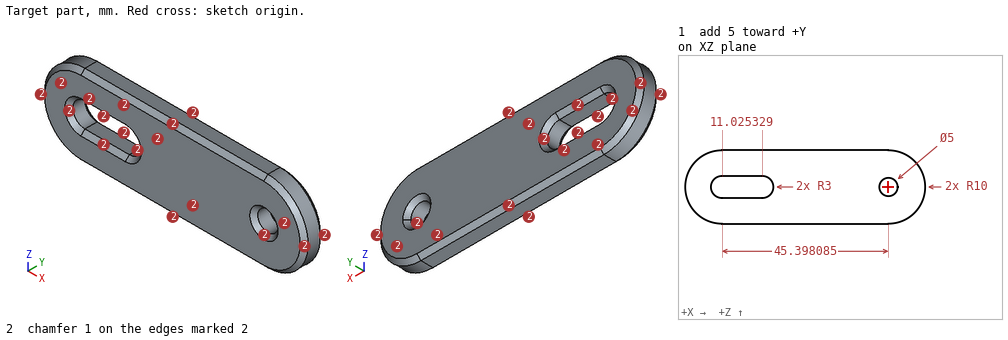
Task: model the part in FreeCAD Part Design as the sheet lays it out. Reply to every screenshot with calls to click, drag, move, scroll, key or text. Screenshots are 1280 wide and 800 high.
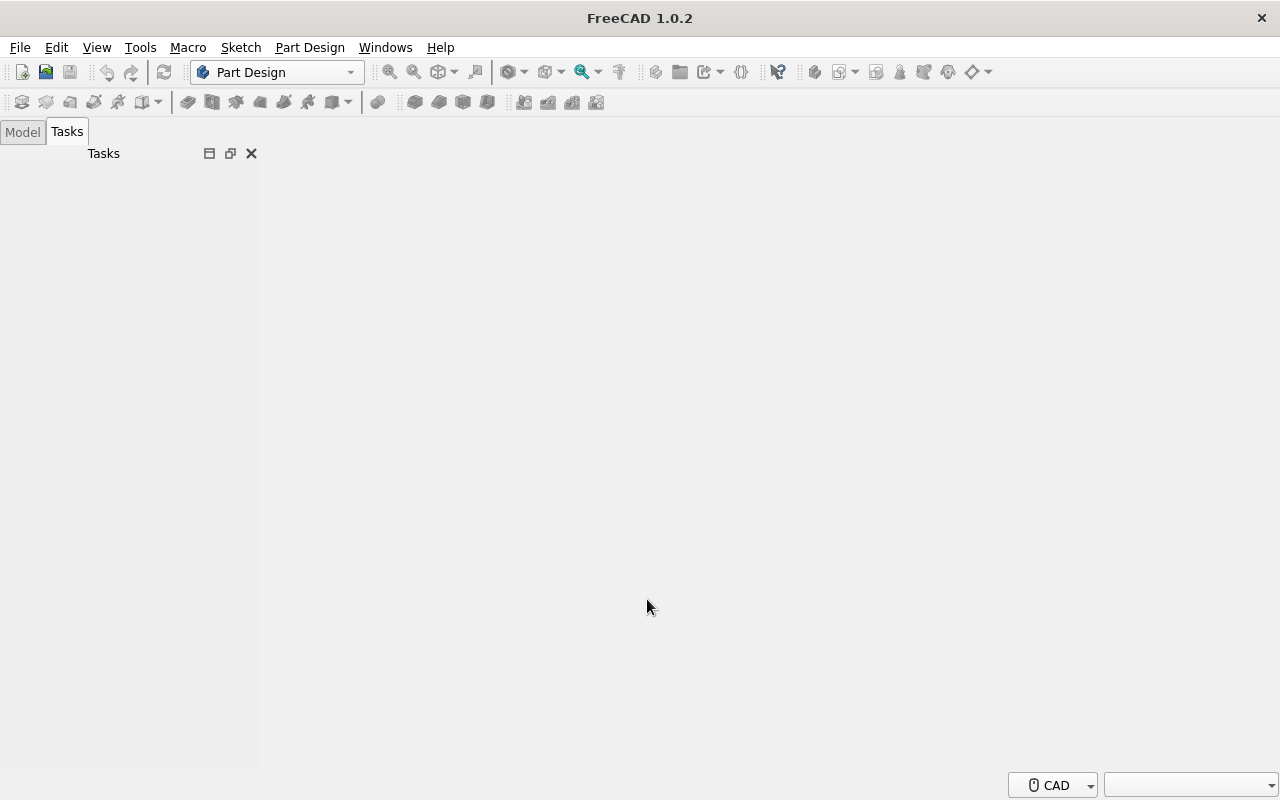
click(22, 72)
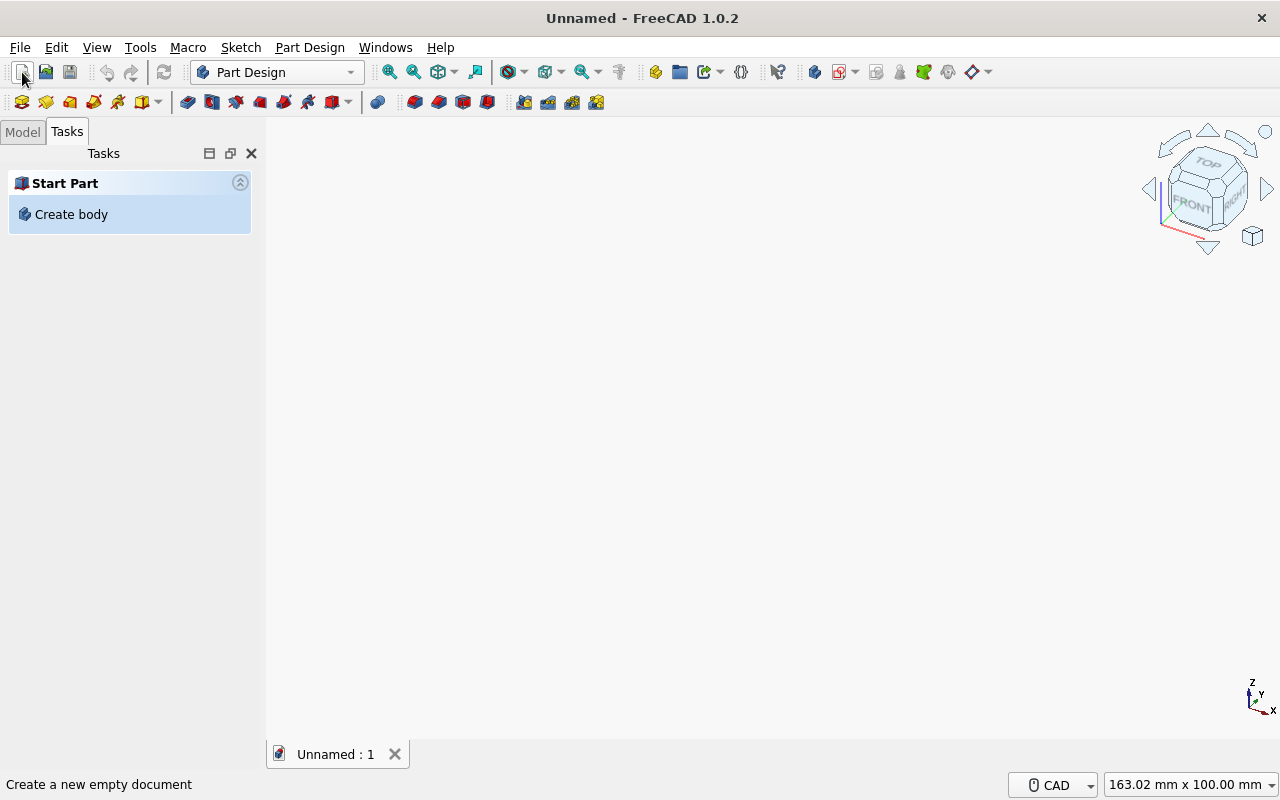
click(840, 72)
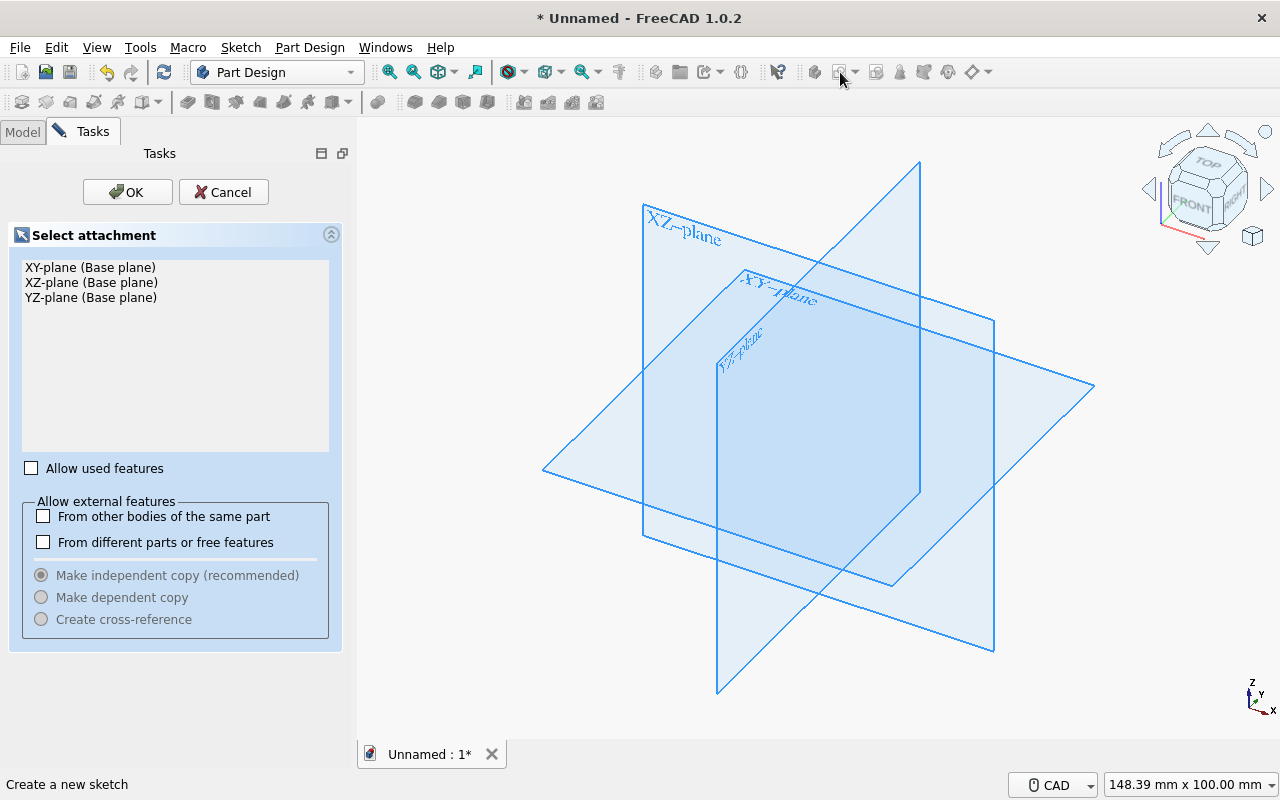
click(82, 282)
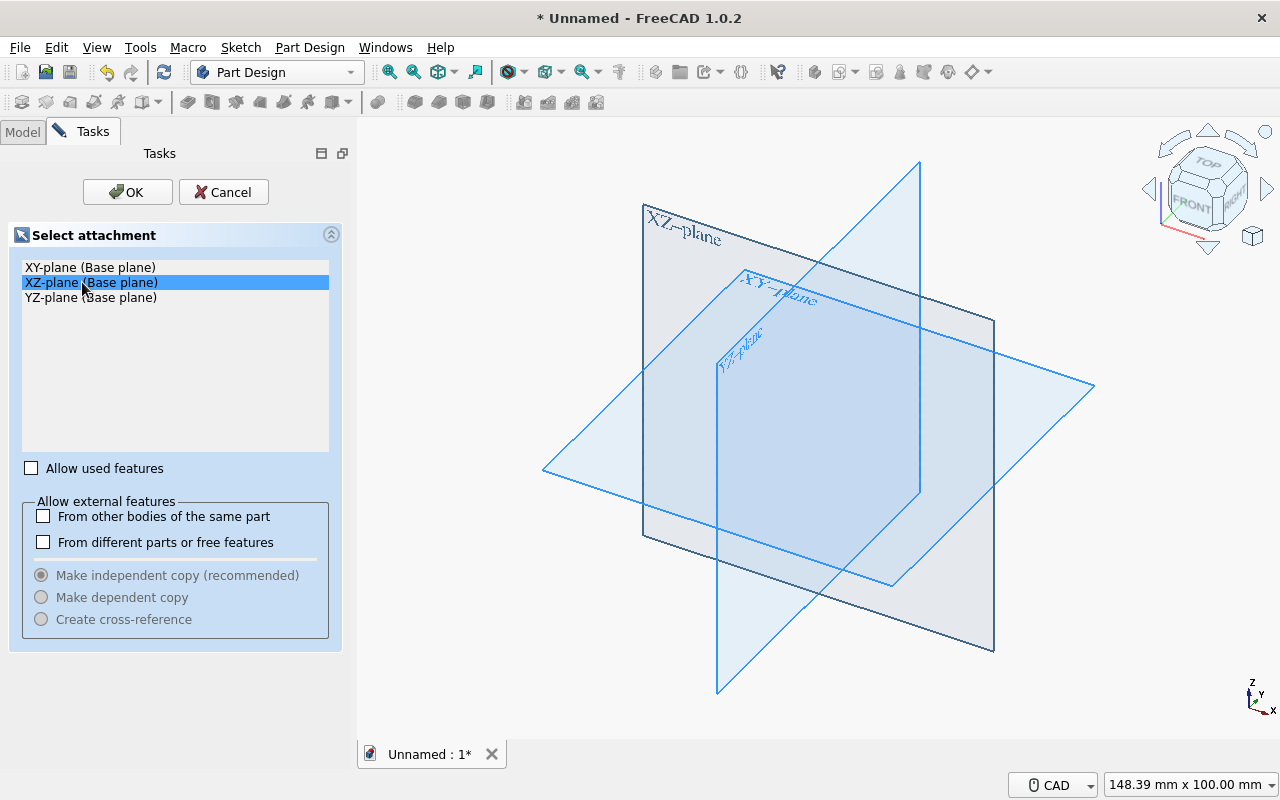
click(128, 192)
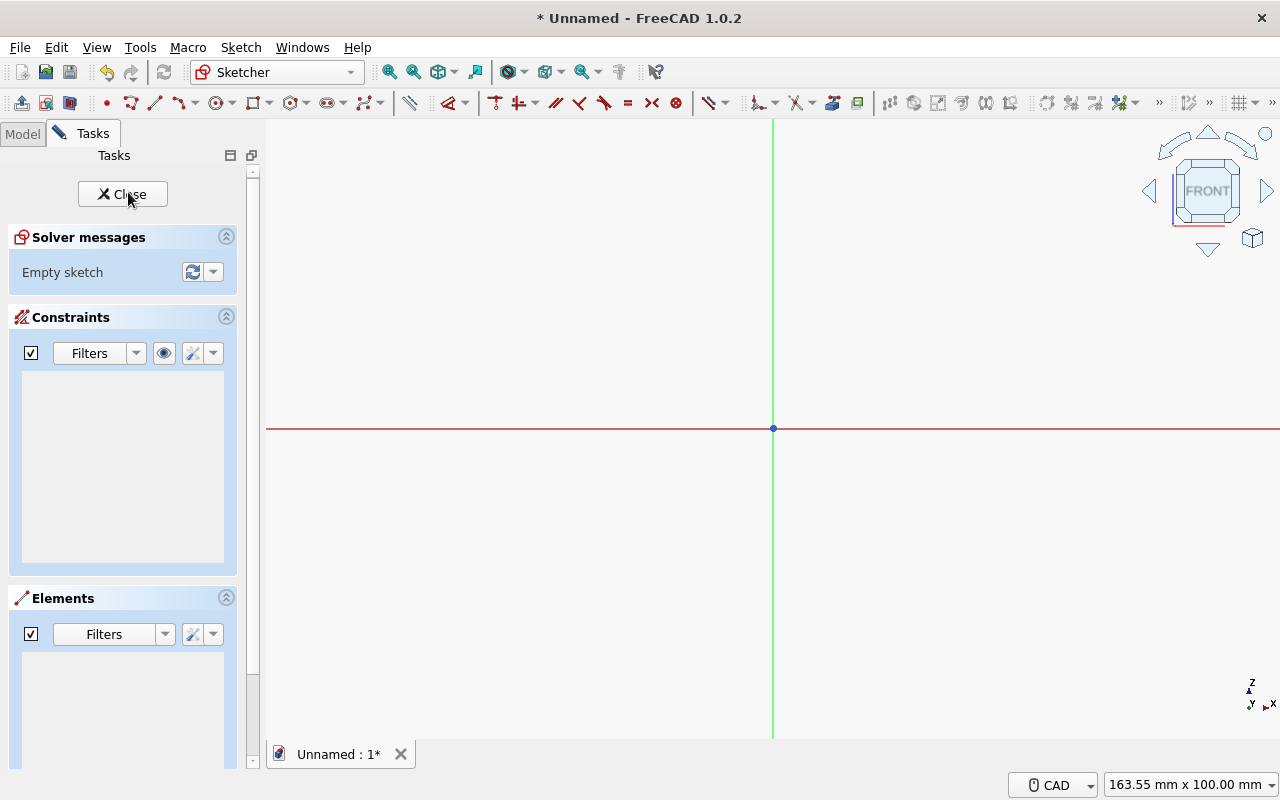
scroll(485, 429, up, 2)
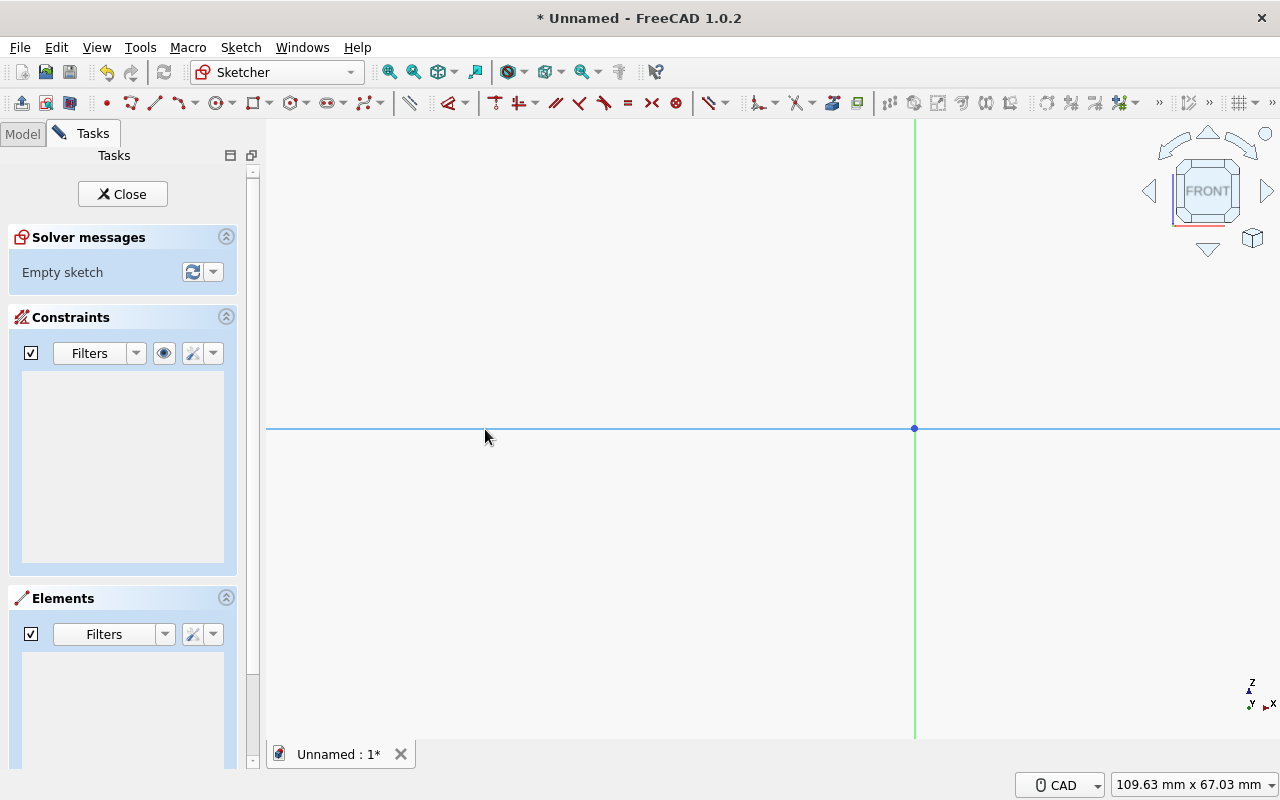
click(328, 104)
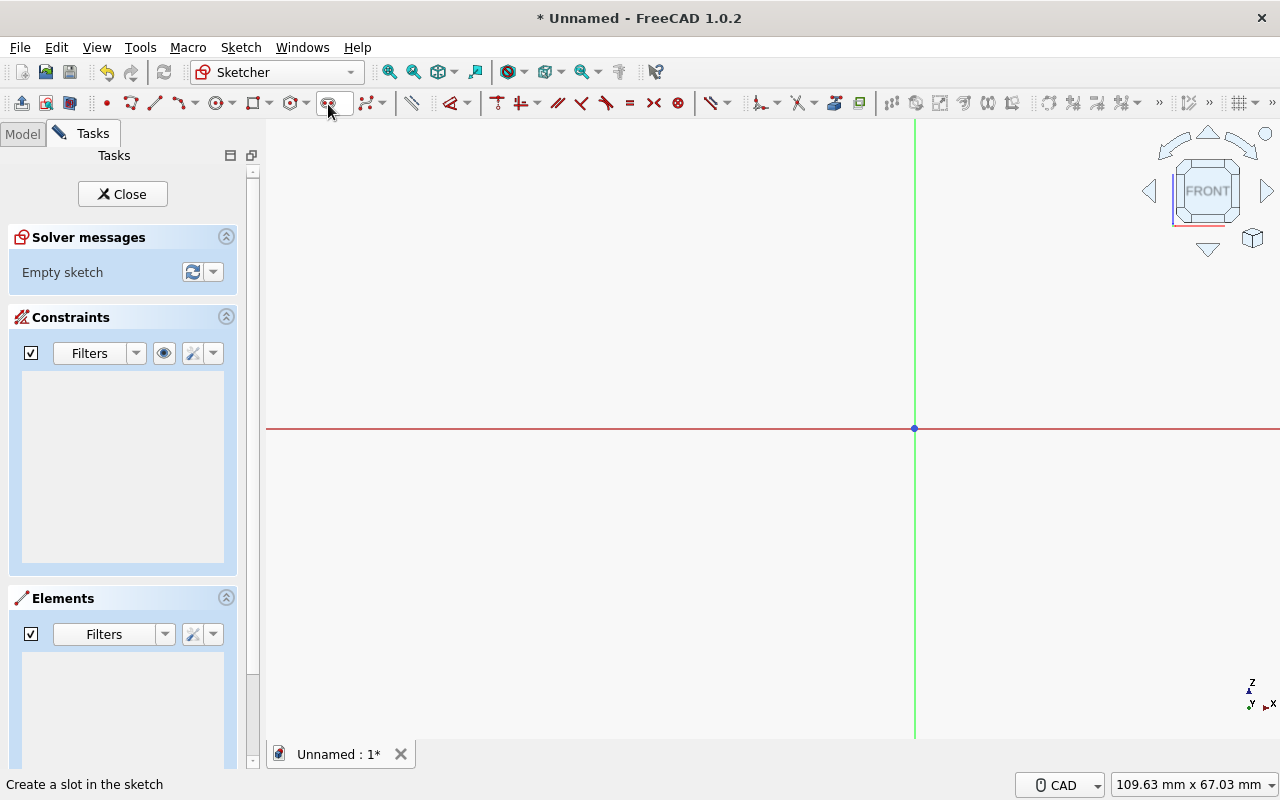
click(915, 429)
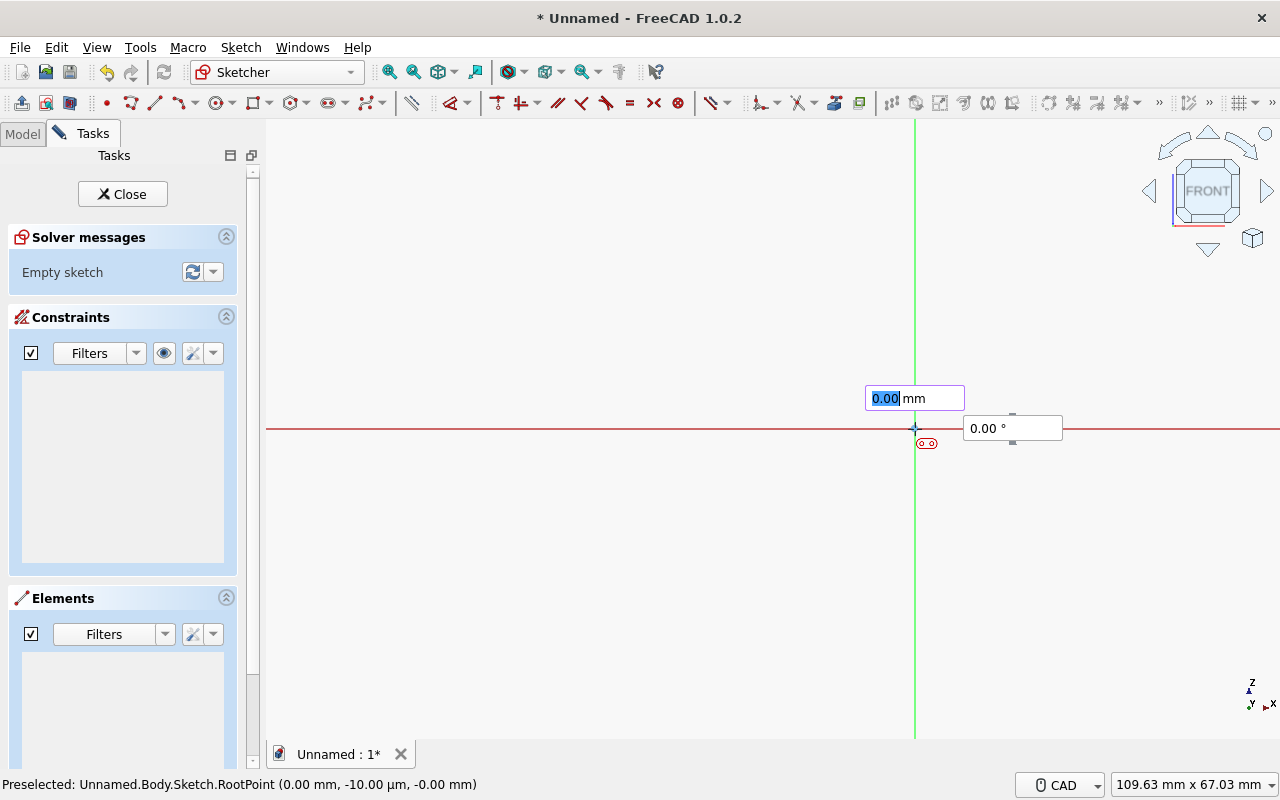
click(495, 420)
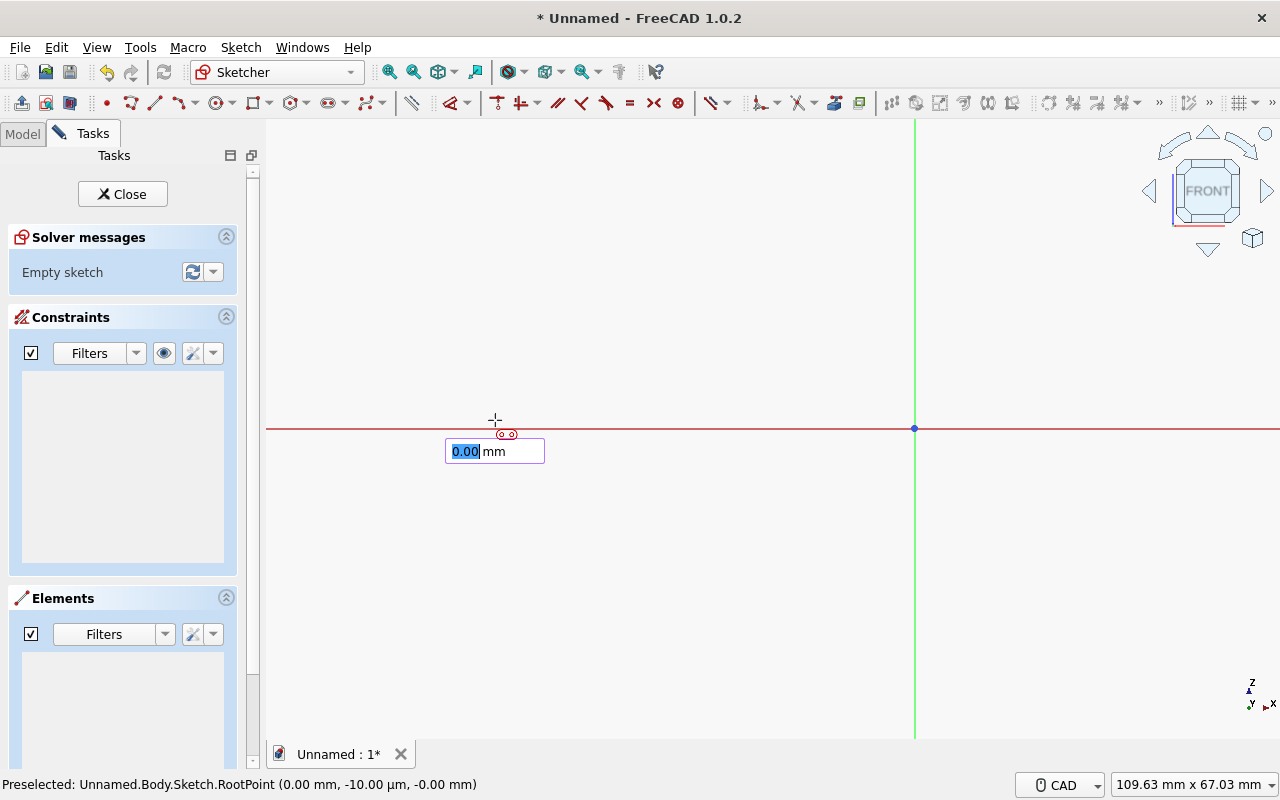
click(705, 336)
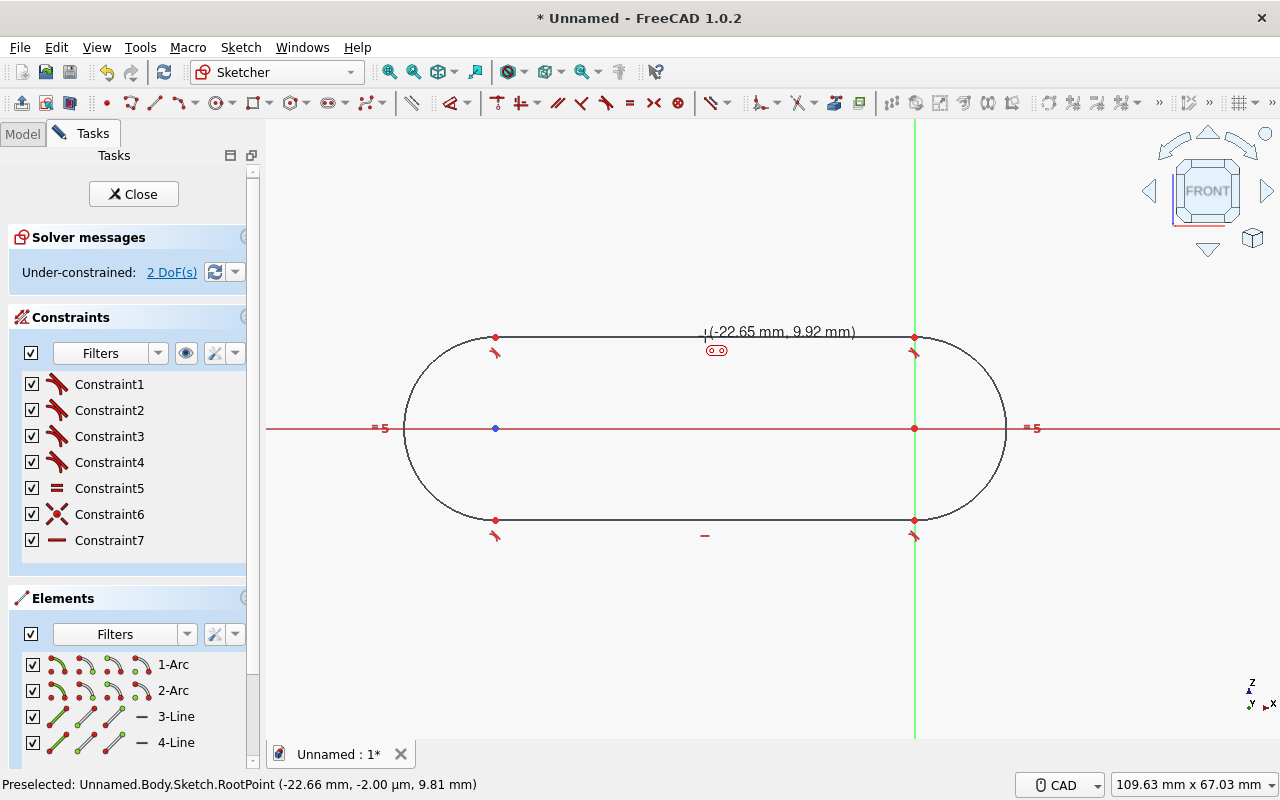
click(496, 429)